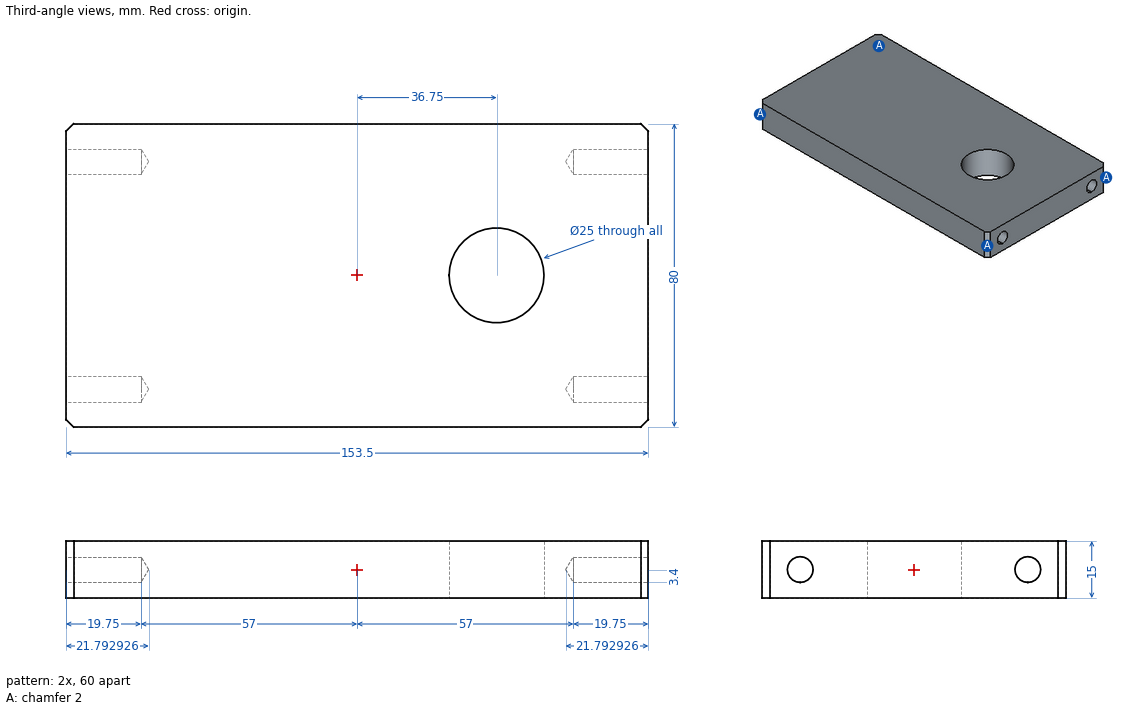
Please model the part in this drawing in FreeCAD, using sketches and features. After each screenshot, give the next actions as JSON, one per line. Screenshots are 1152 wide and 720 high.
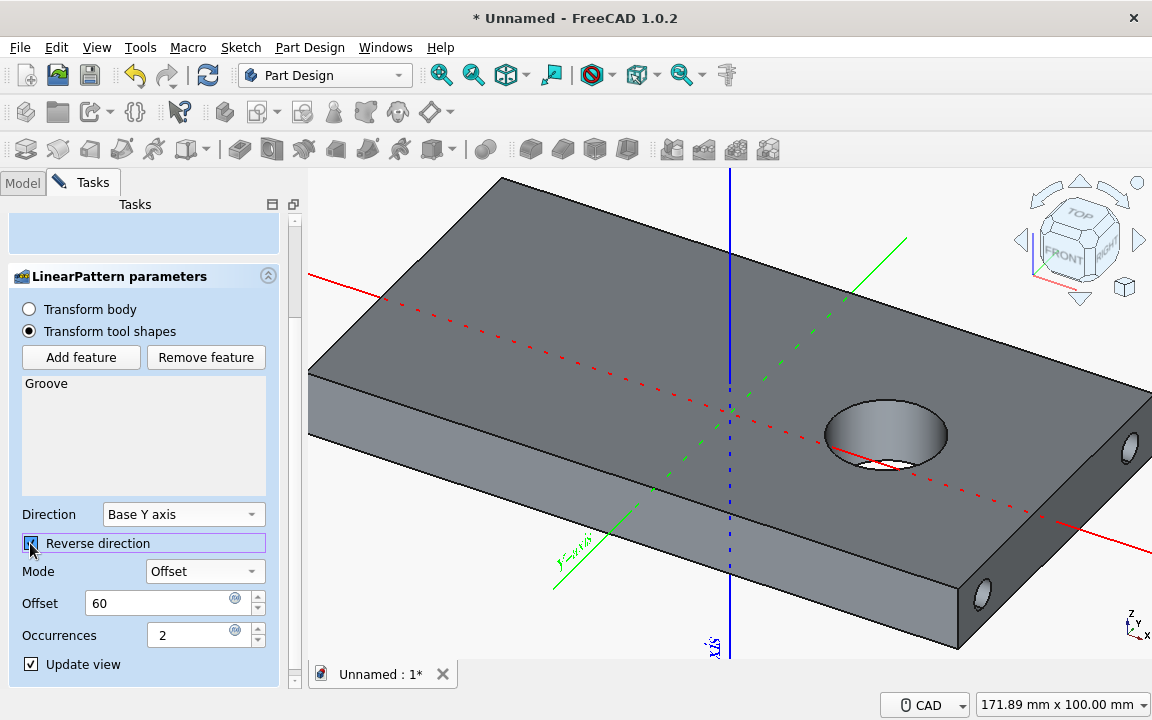
{"action": "scroll", "coordinate": [295, 451], "scroll_direction": "up", "scroll_amount": 3}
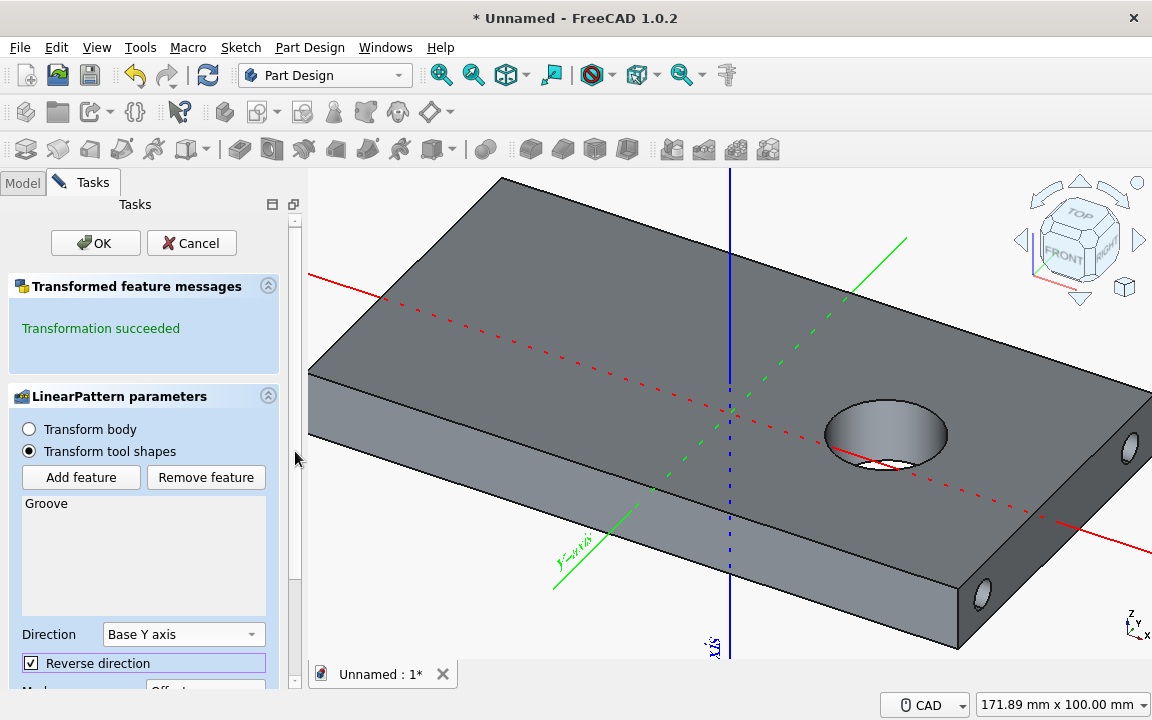
{"action": "left_click", "coordinate": [96, 243]}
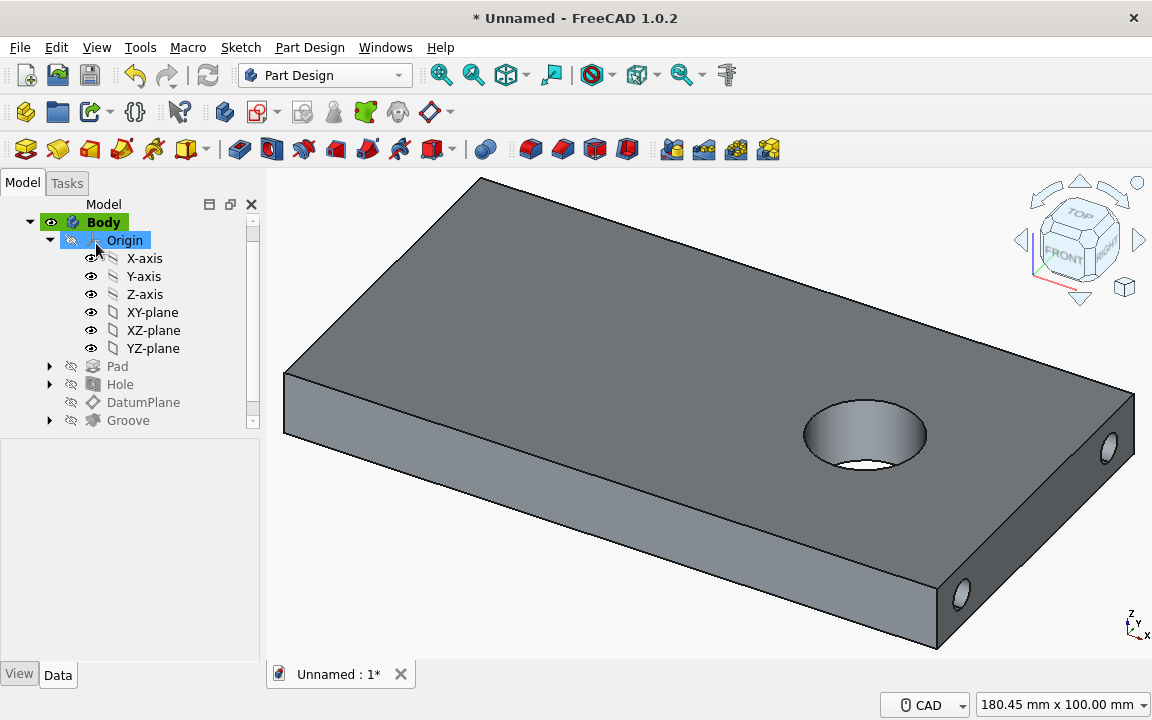
{"action": "left_click", "coordinate": [116, 420]}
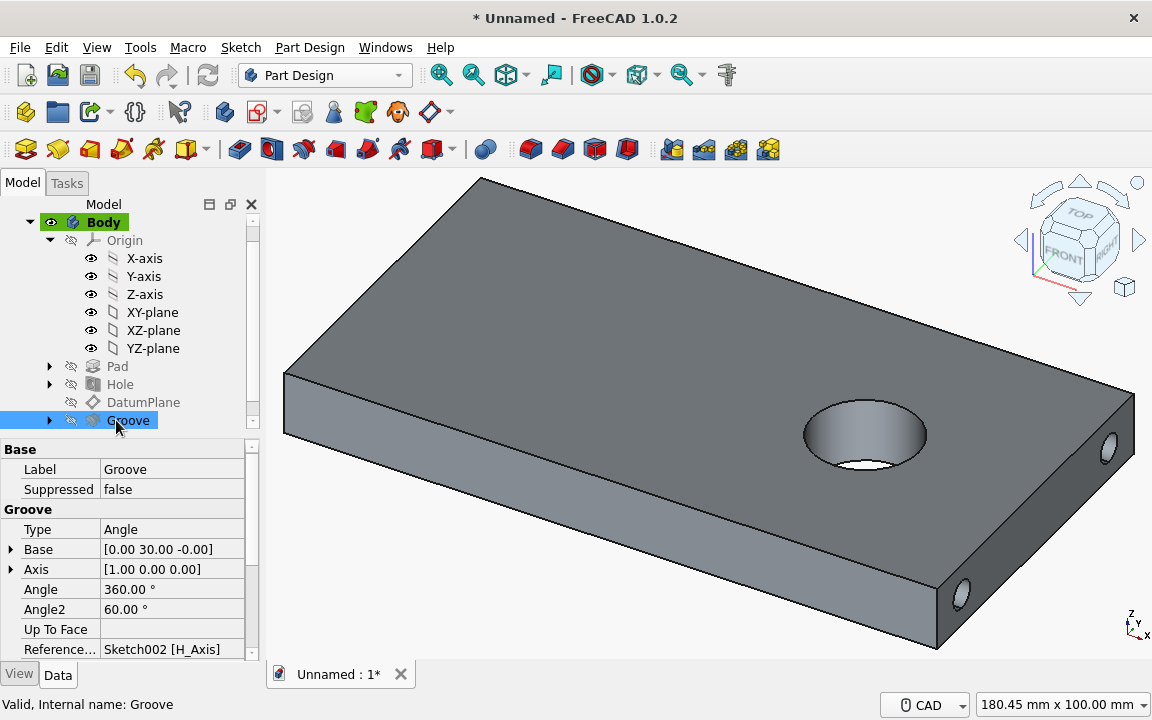
{"action": "left_click", "coordinate": [672, 150]}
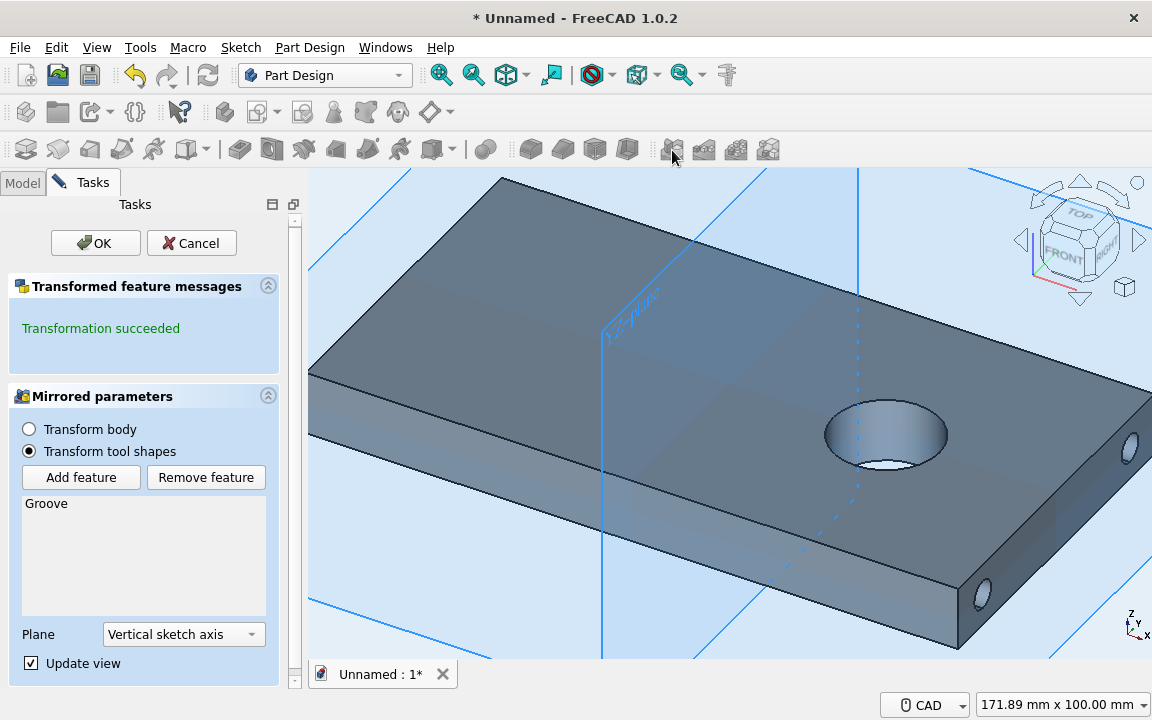
{"action": "left_click", "coordinate": [184, 634]}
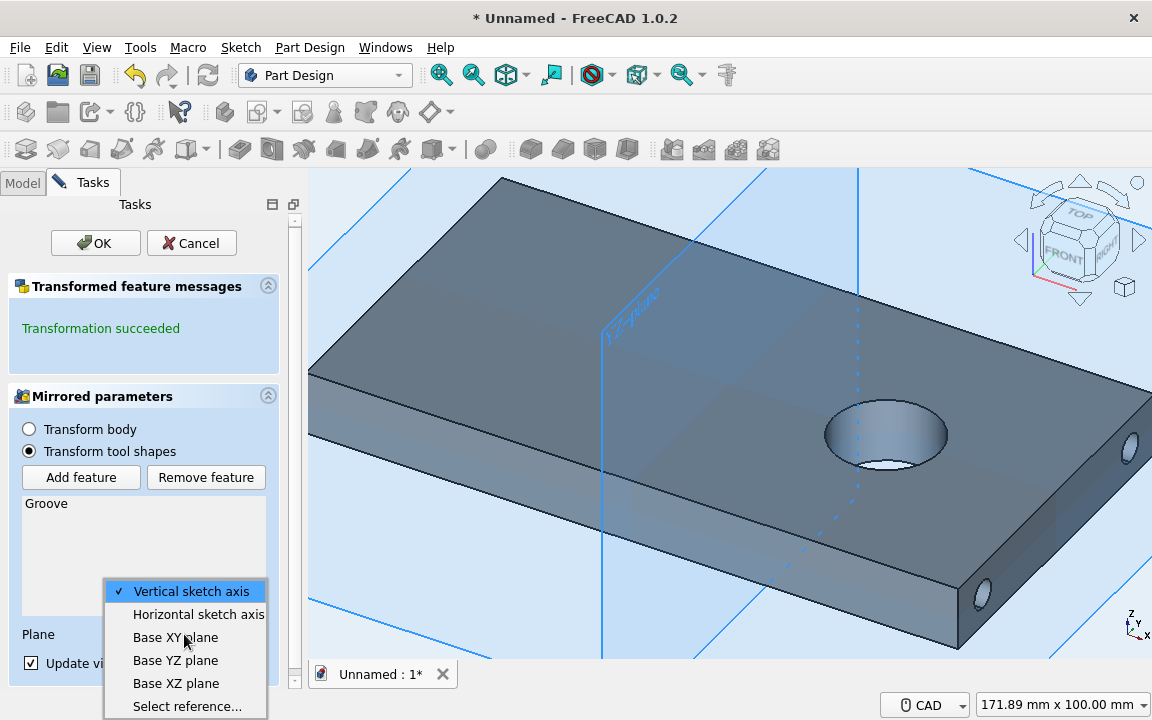
{"action": "left_click", "coordinate": [184, 660]}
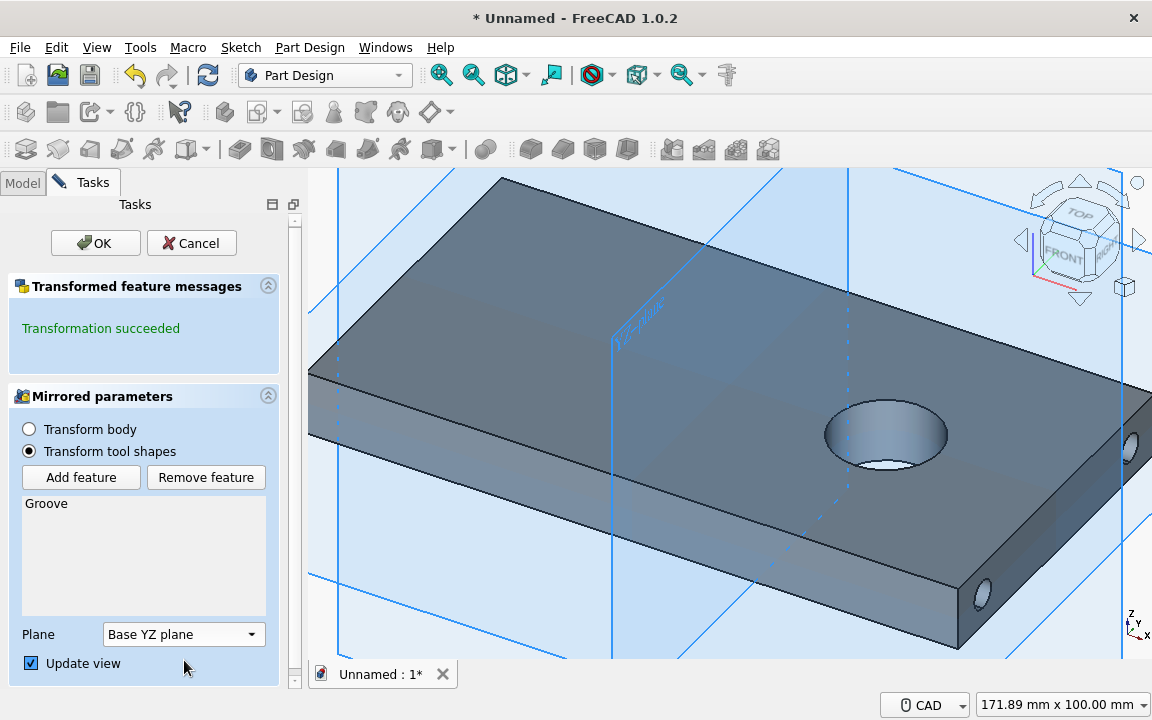
{"action": "left_click", "coordinate": [96, 243]}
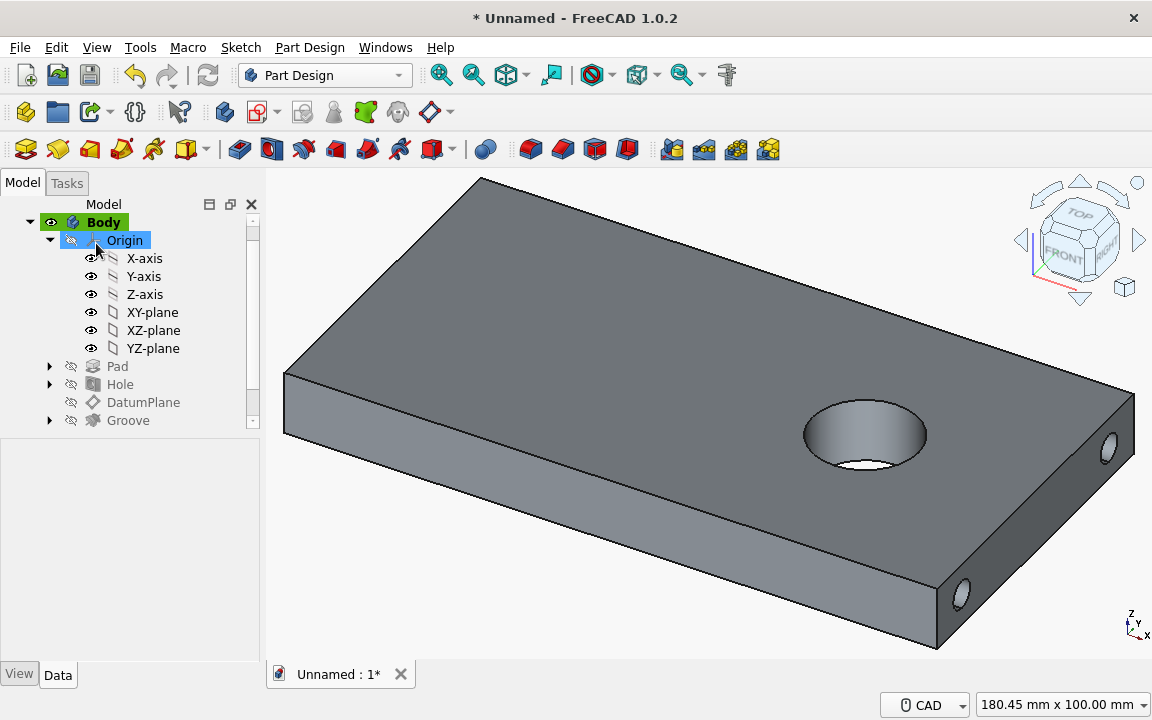
{"action": "left_click", "coordinate": [136, 330]}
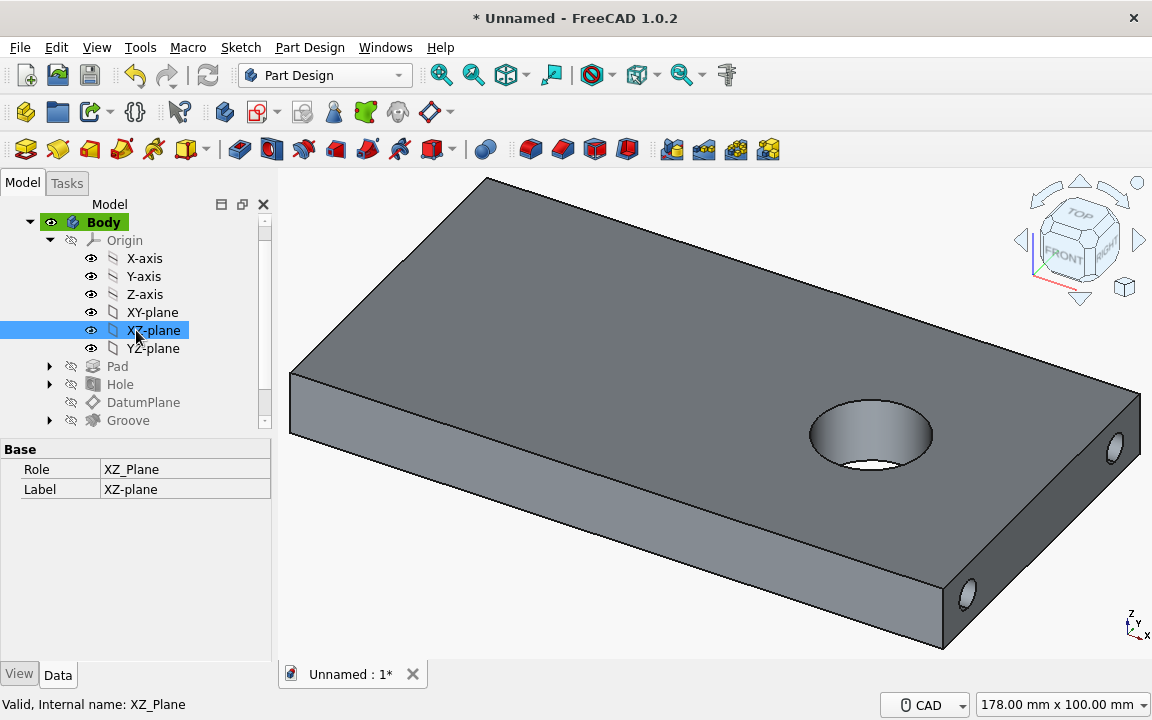
{"action": "left_click", "coordinate": [430, 112]}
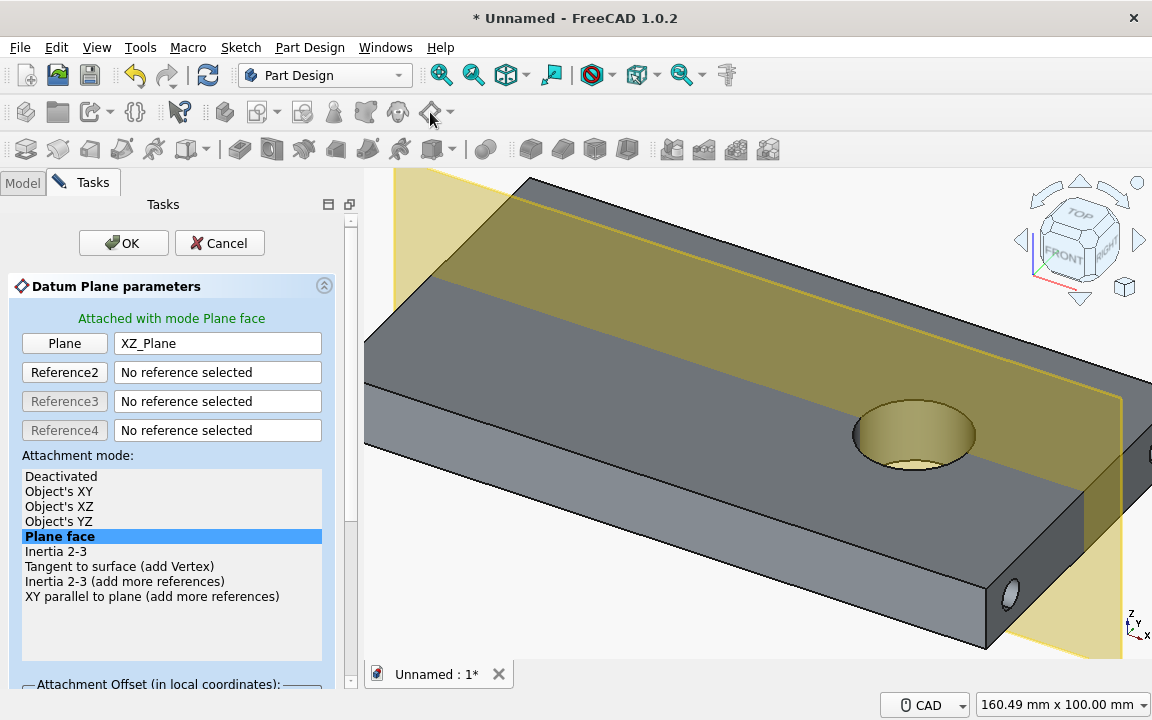
{"action": "scroll", "coordinate": [351, 451], "scroll_direction": "down", "scroll_amount": 3}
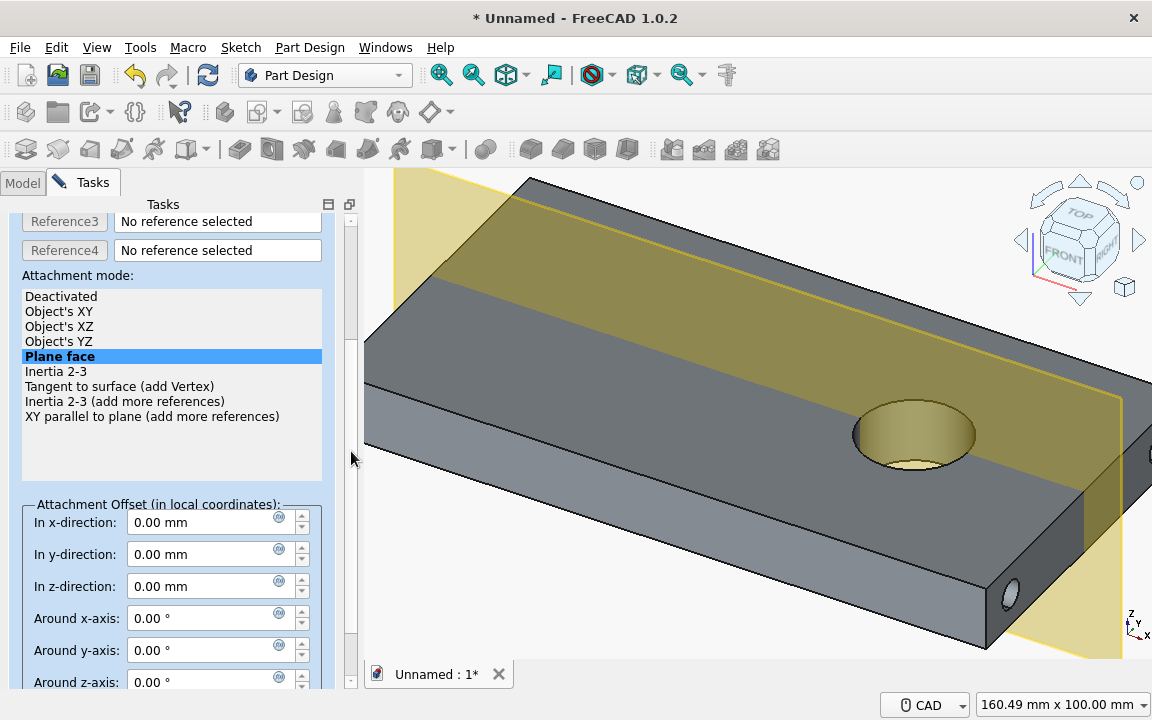
{"action": "triple_click", "coordinate": [210, 586]}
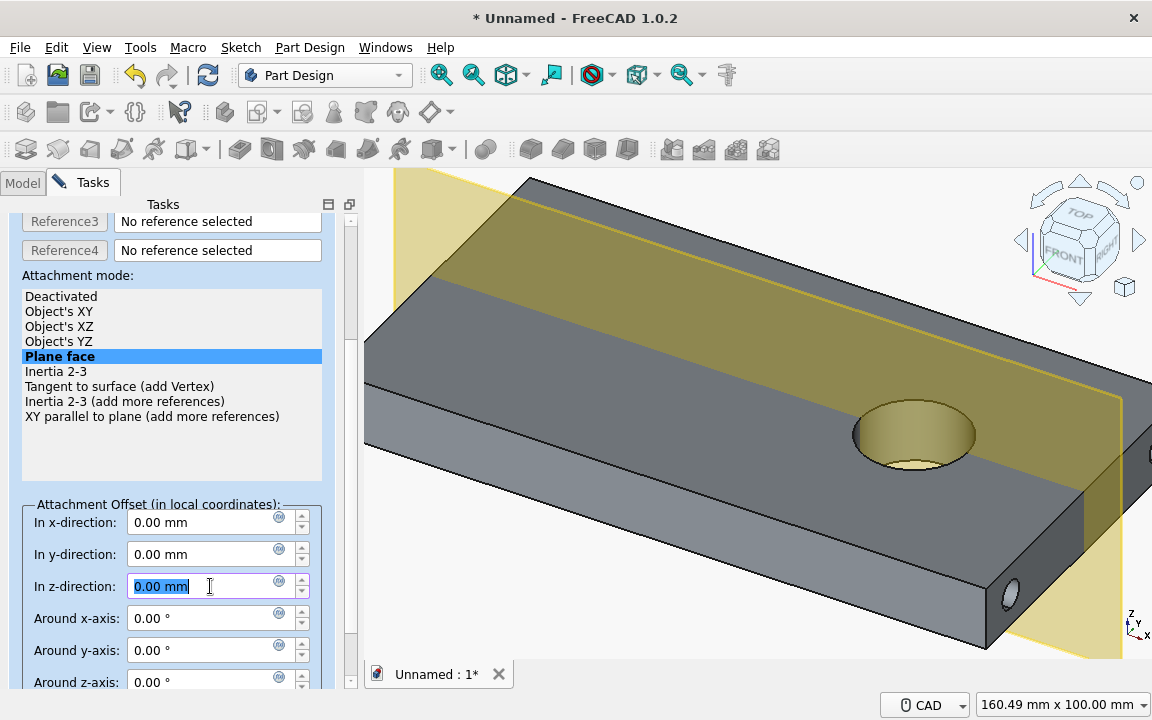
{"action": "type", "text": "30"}
{"action": "key", "text": "Tab"}